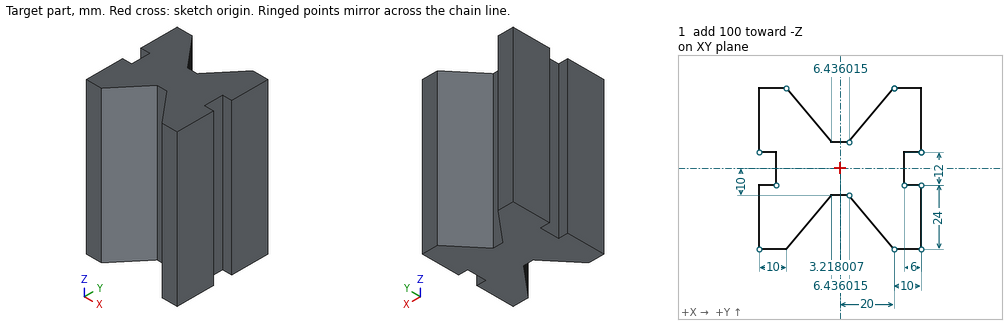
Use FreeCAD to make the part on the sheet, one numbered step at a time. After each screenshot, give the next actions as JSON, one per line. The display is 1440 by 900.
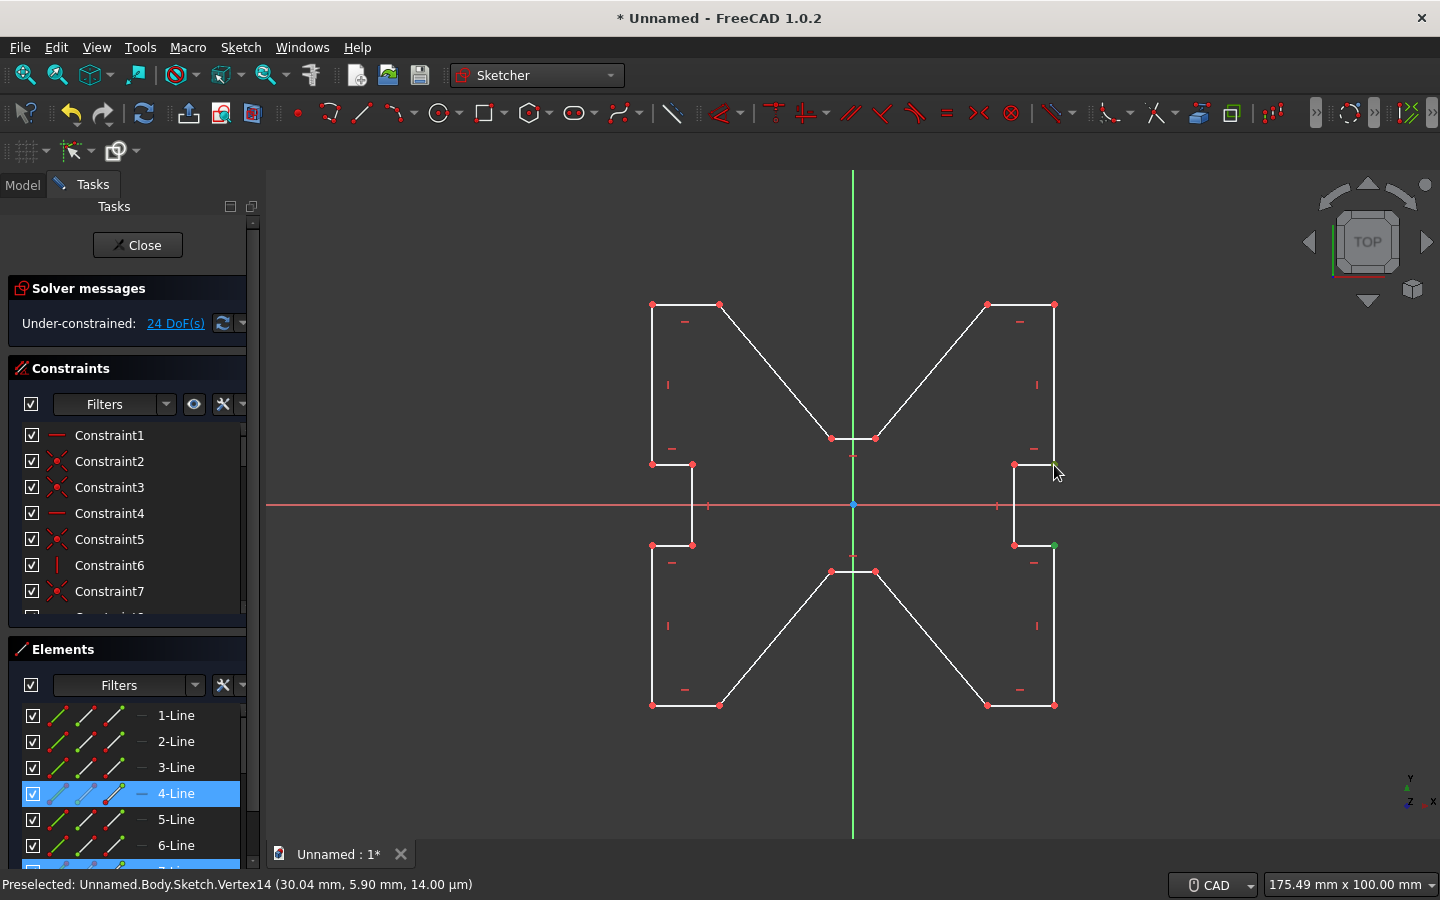
{"action": "left_click", "coordinate": [364, 504]}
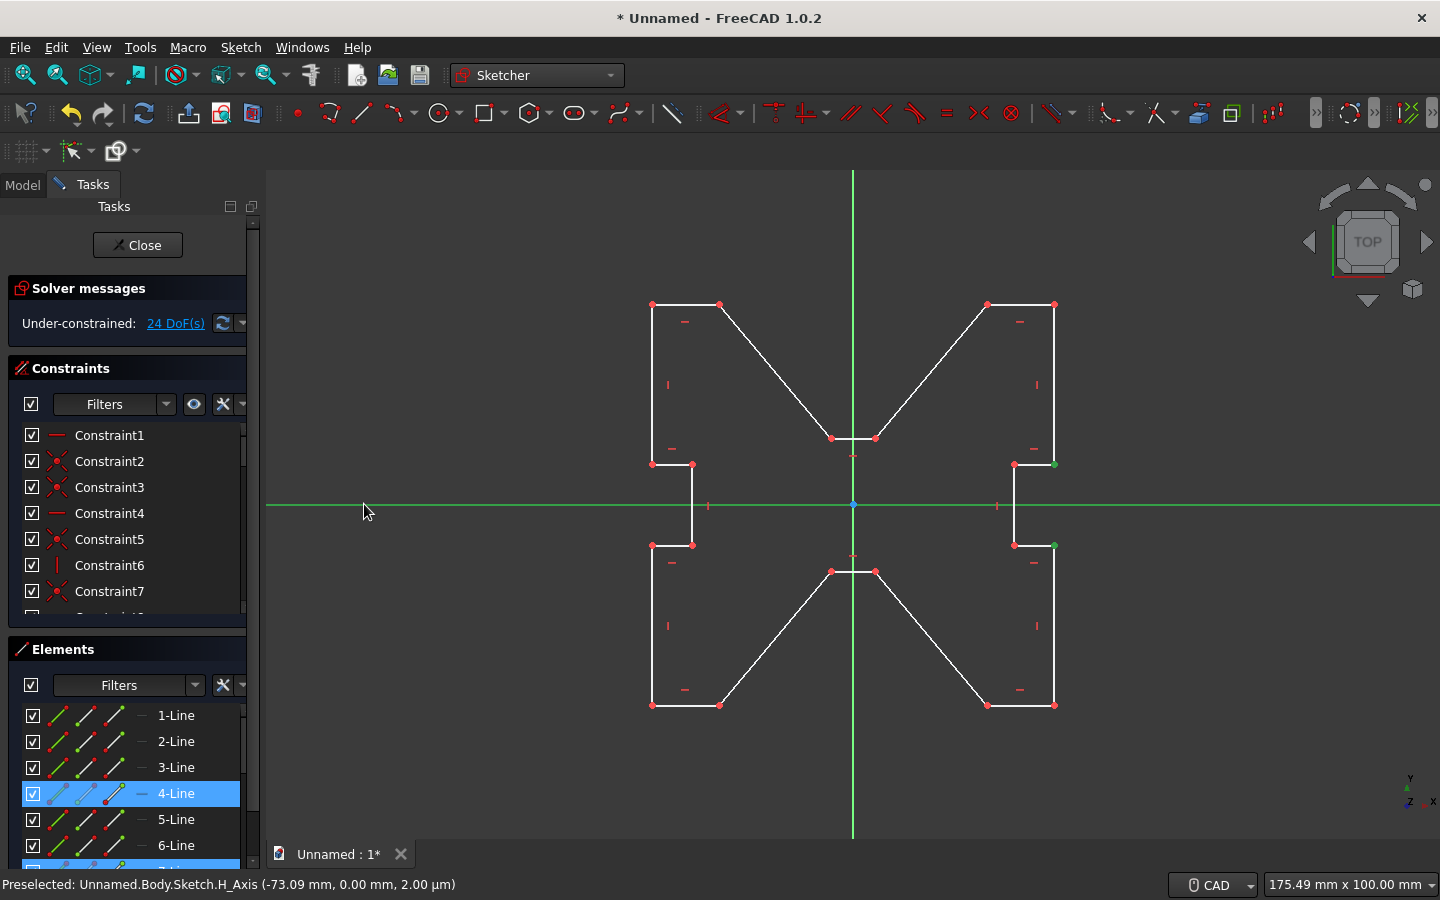
{"action": "key", "text": "s"}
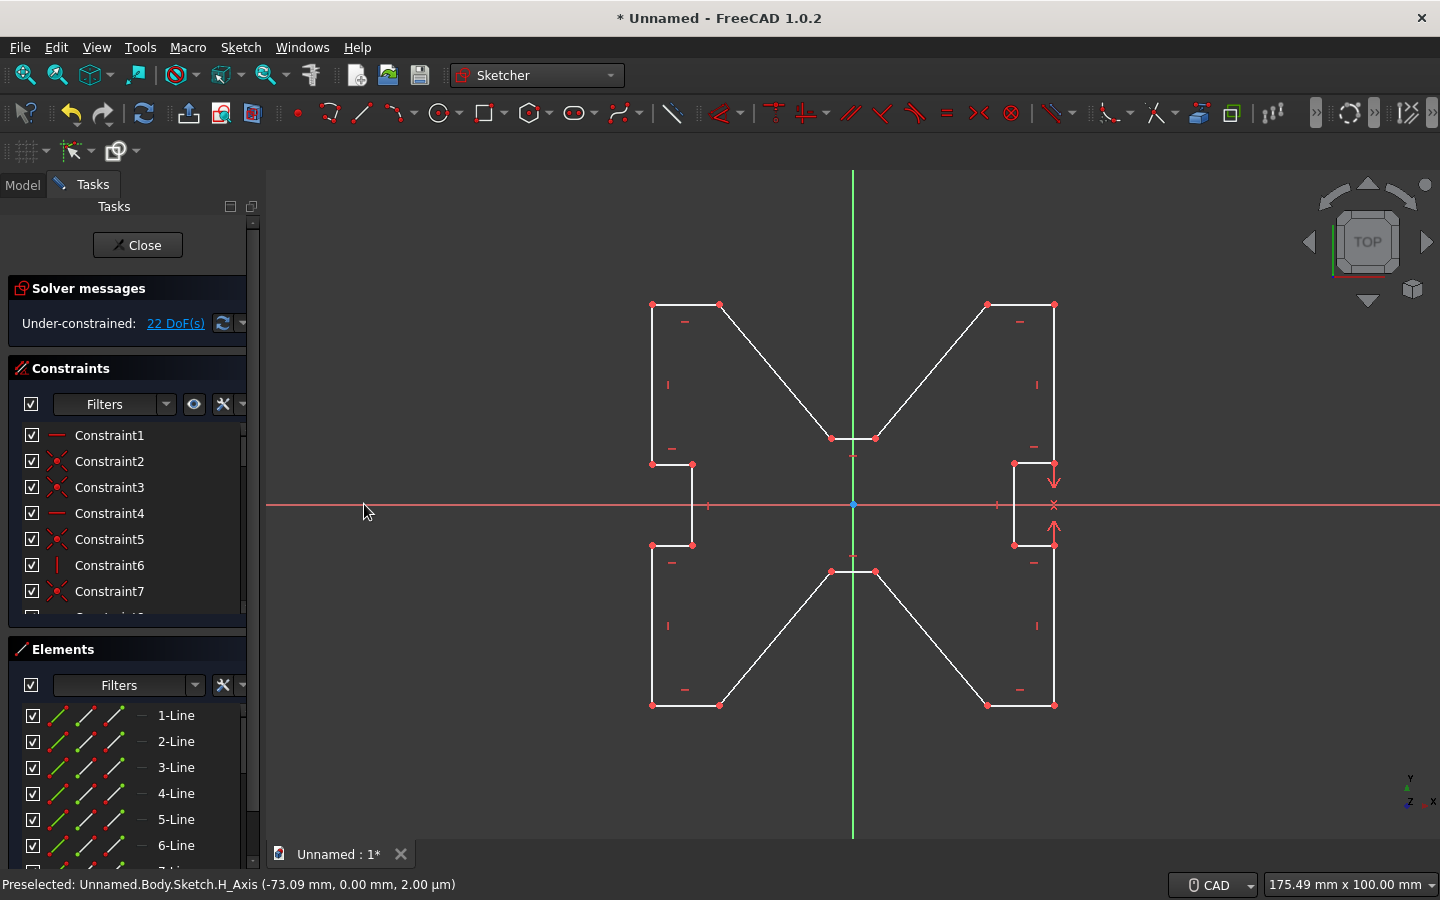
{"action": "left_click", "coordinate": [987, 706]}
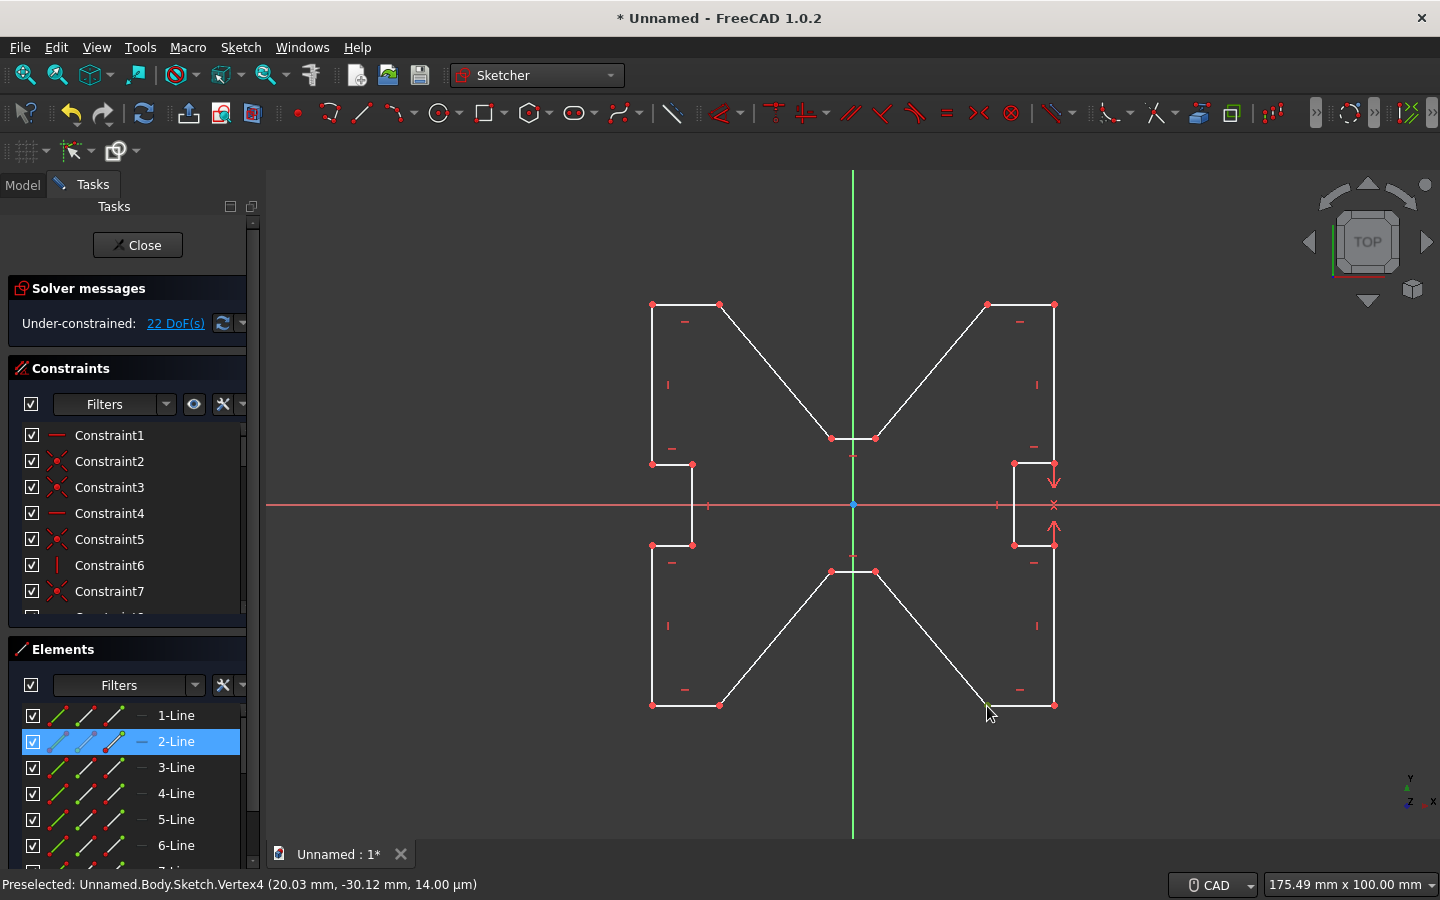
{"action": "left_click", "coordinate": [987, 305]}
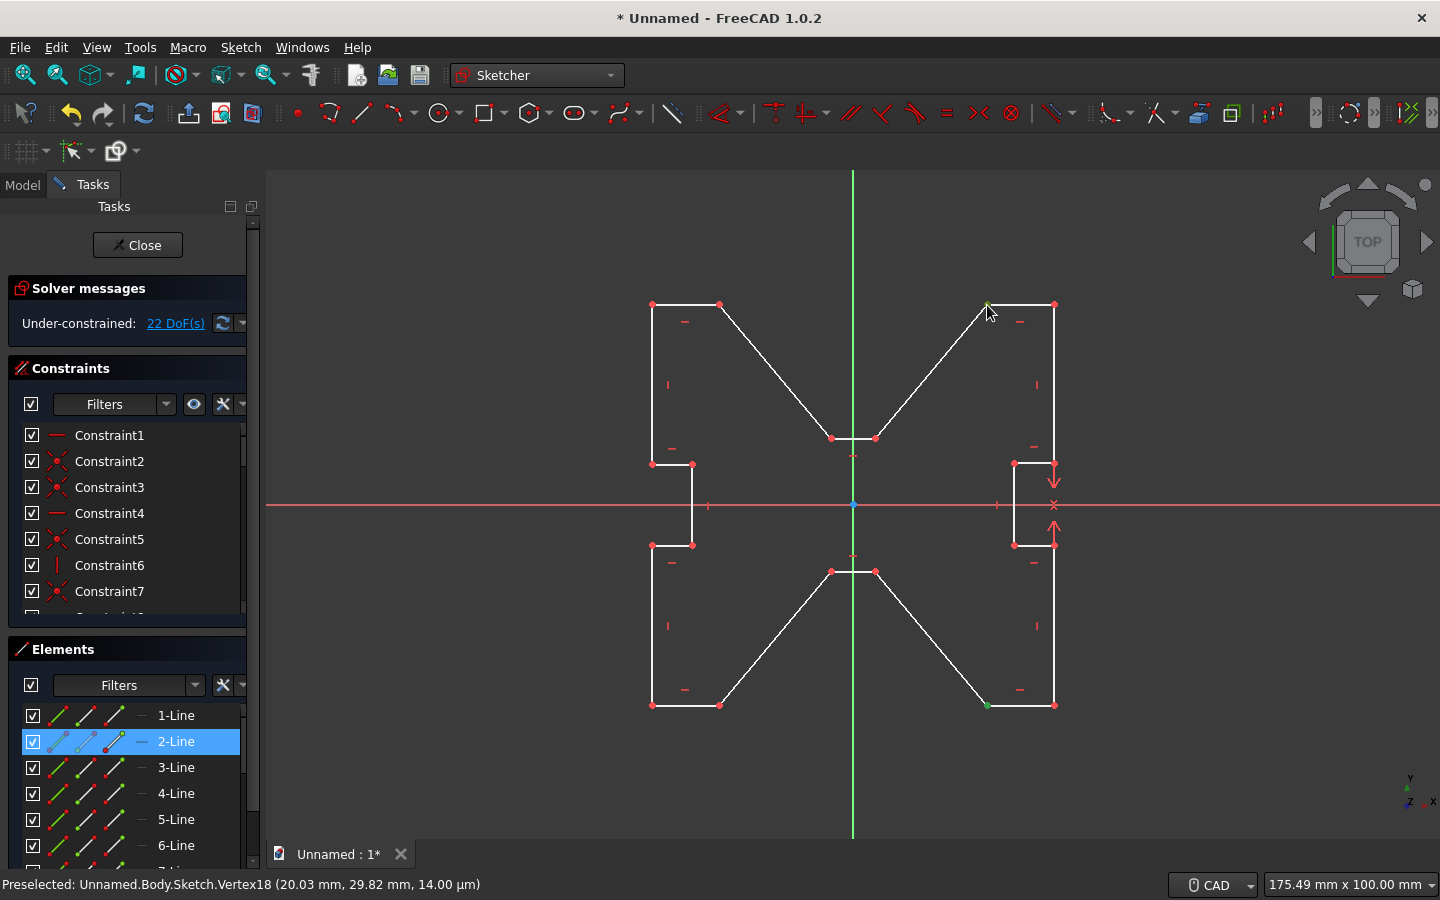
{"action": "left_click", "coordinate": [364, 504]}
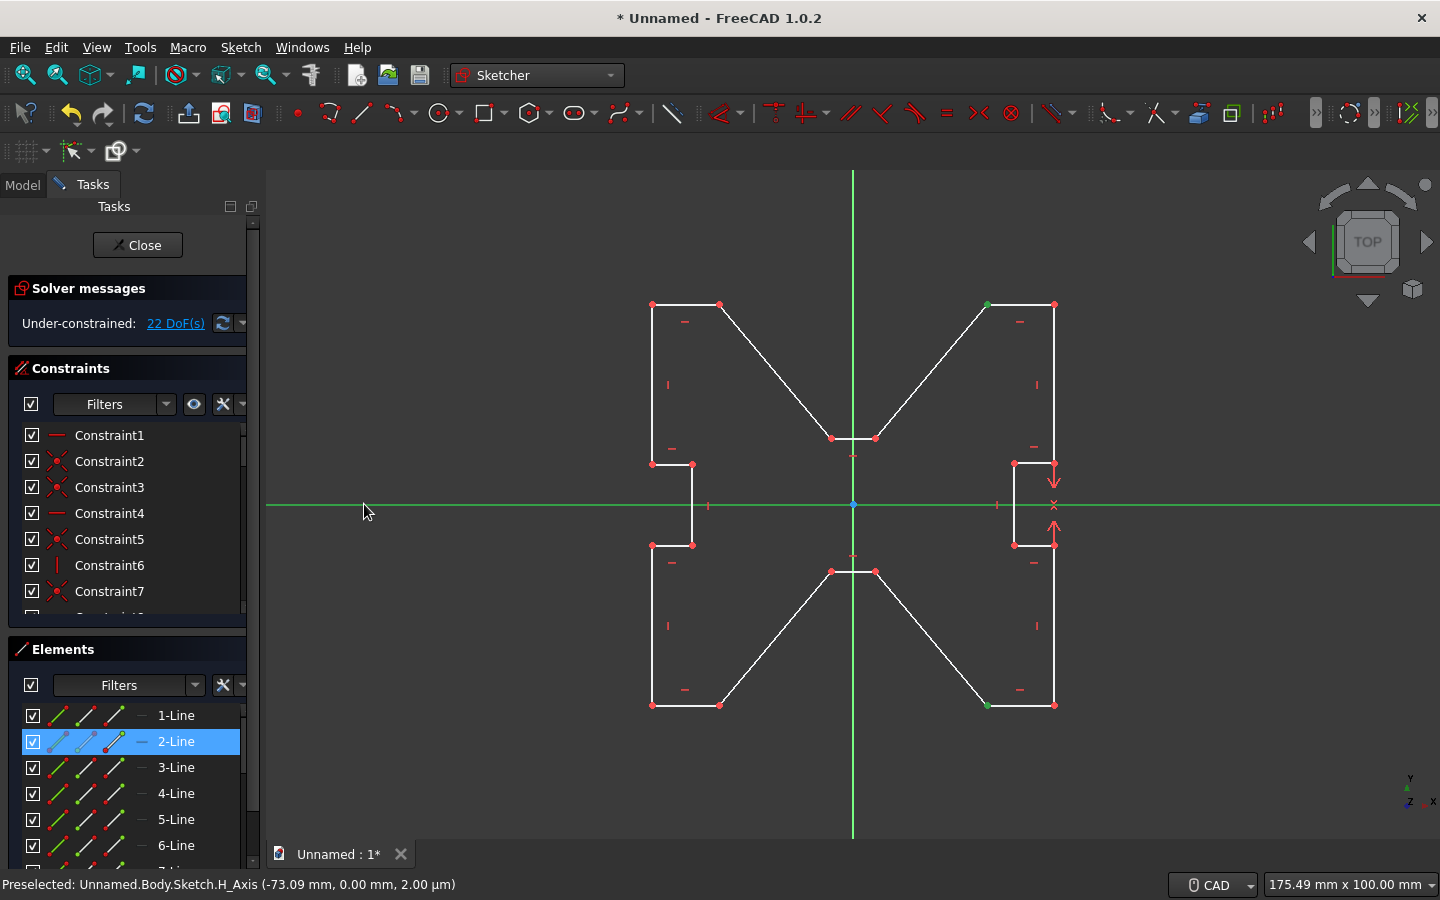
{"action": "key", "text": "s"}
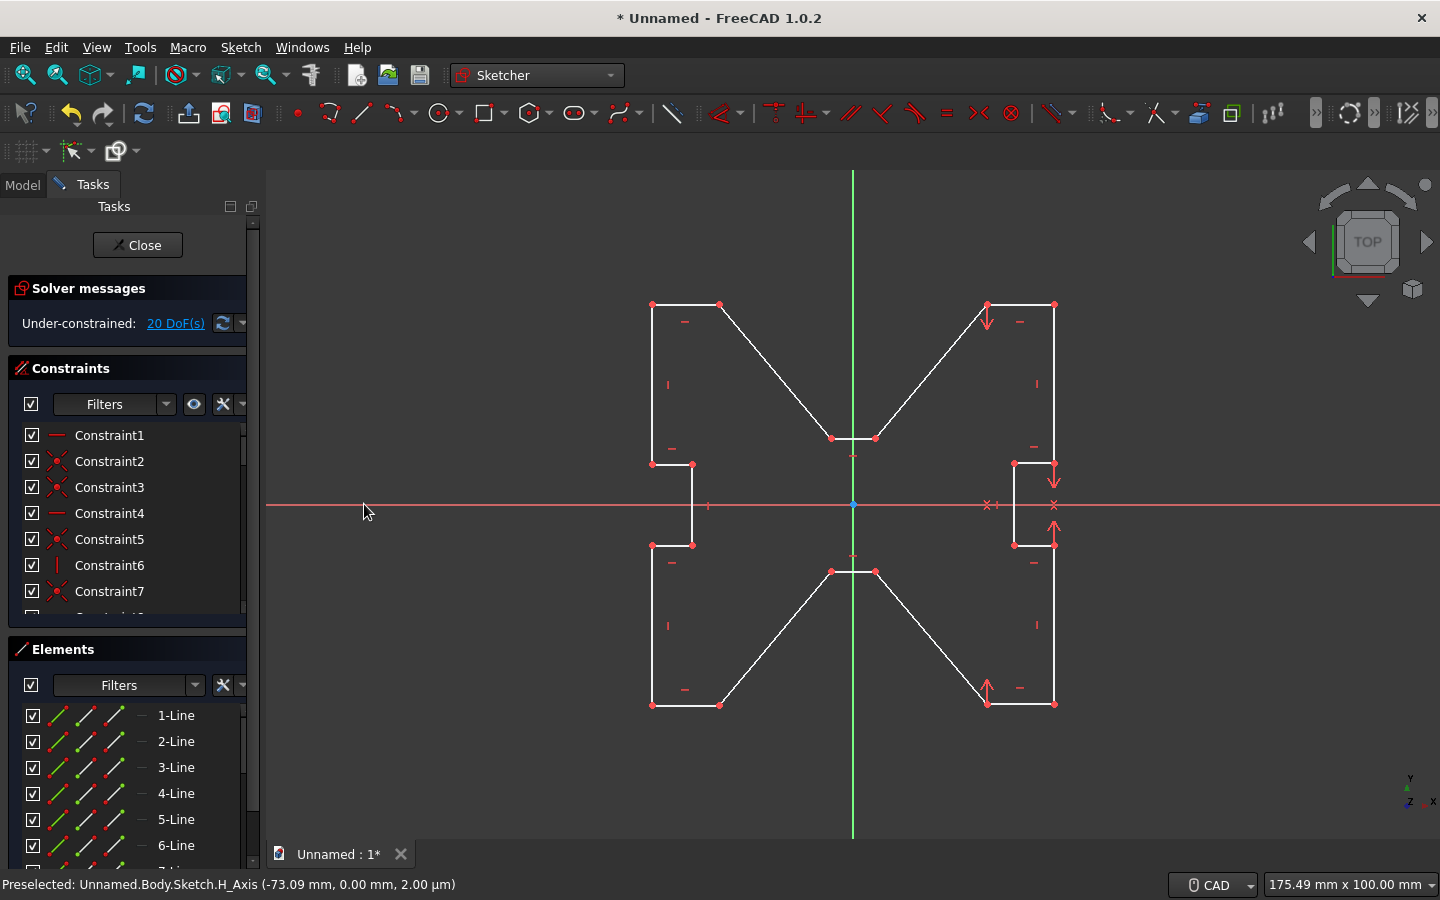
{"action": "left_click", "coordinate": [875, 572]}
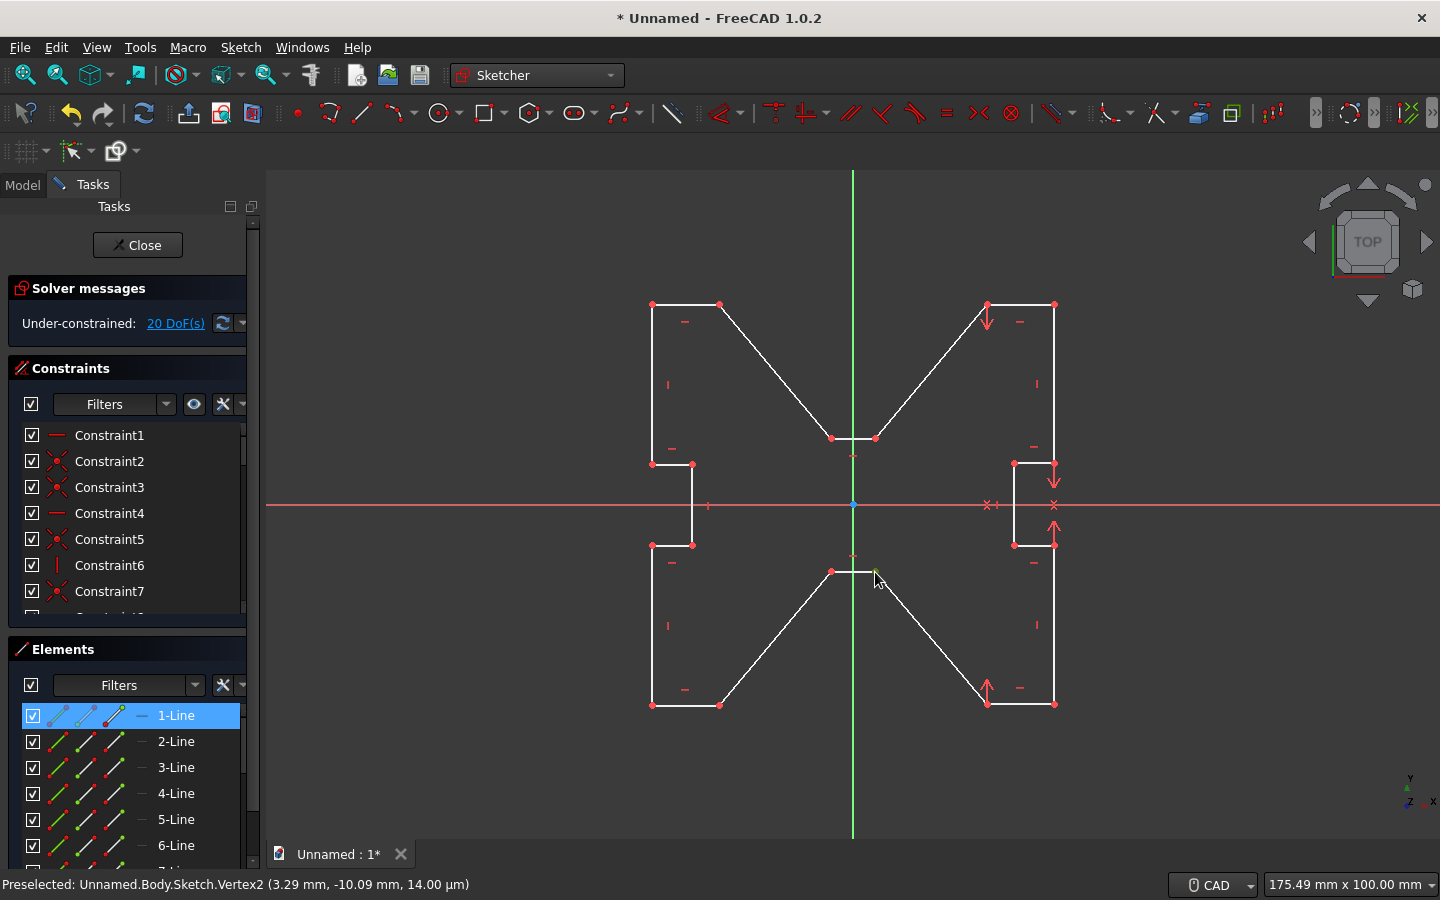
{"action": "left_click", "coordinate": [875, 439]}